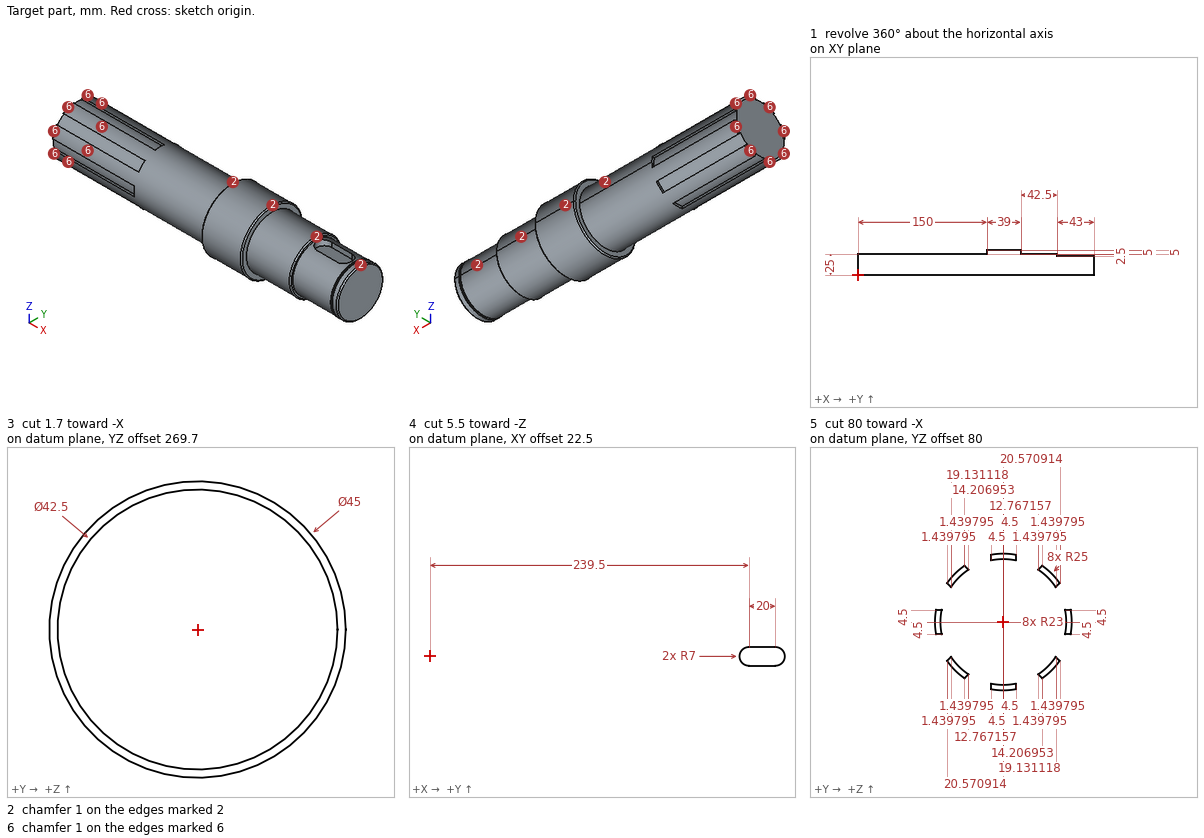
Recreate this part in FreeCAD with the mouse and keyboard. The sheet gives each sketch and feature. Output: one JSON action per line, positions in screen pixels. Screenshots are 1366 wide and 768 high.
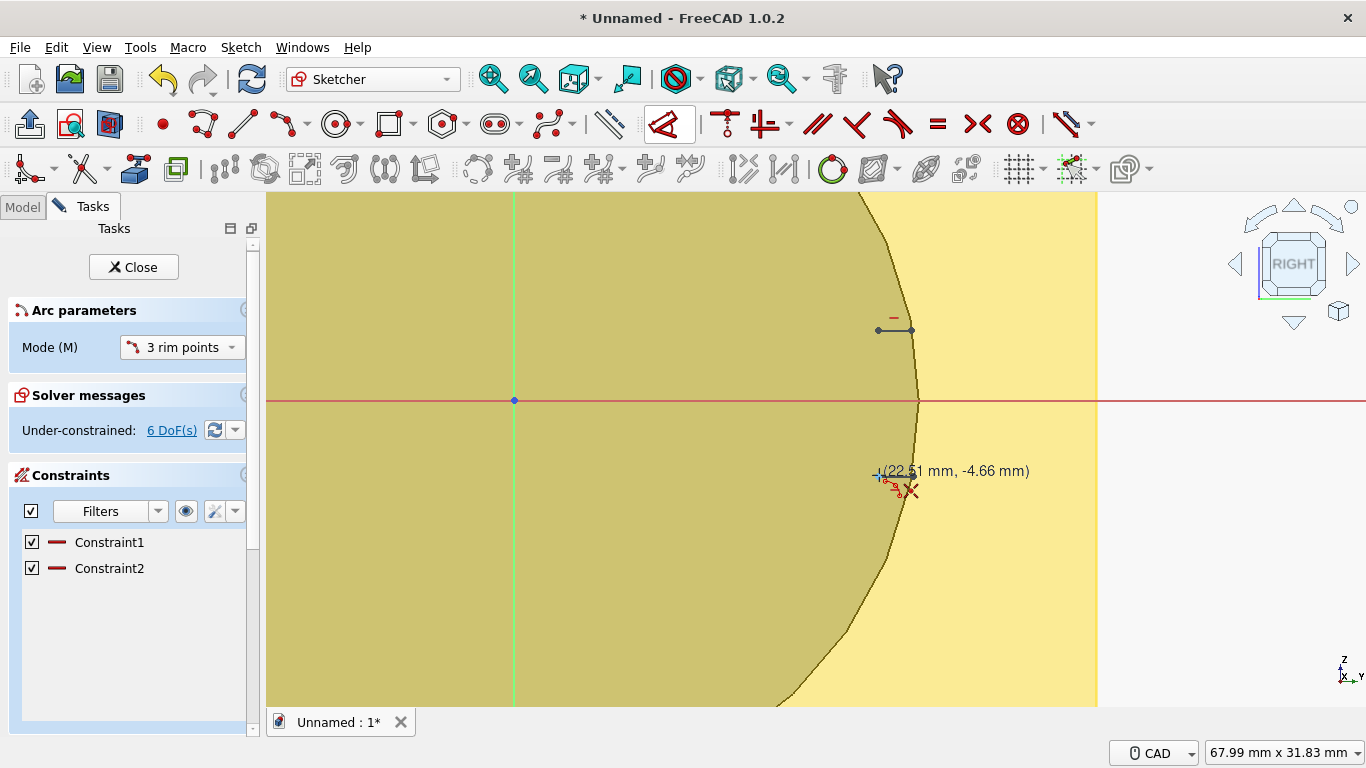
{"action": "left_click", "coordinate": [879, 477]}
{"action": "left_click", "coordinate": [879, 331]}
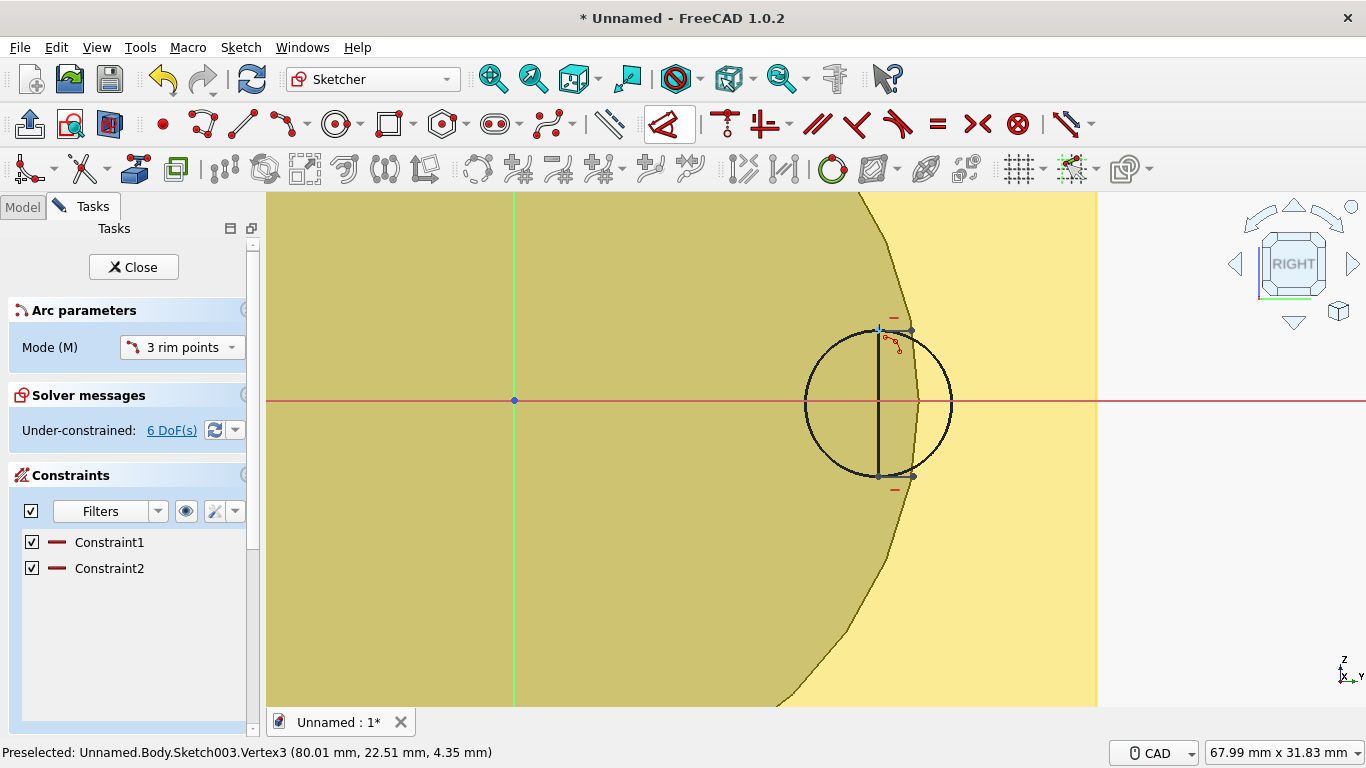
{"action": "scroll", "coordinate": [886, 416], "scroll_direction": "up", "scroll_amount": 5}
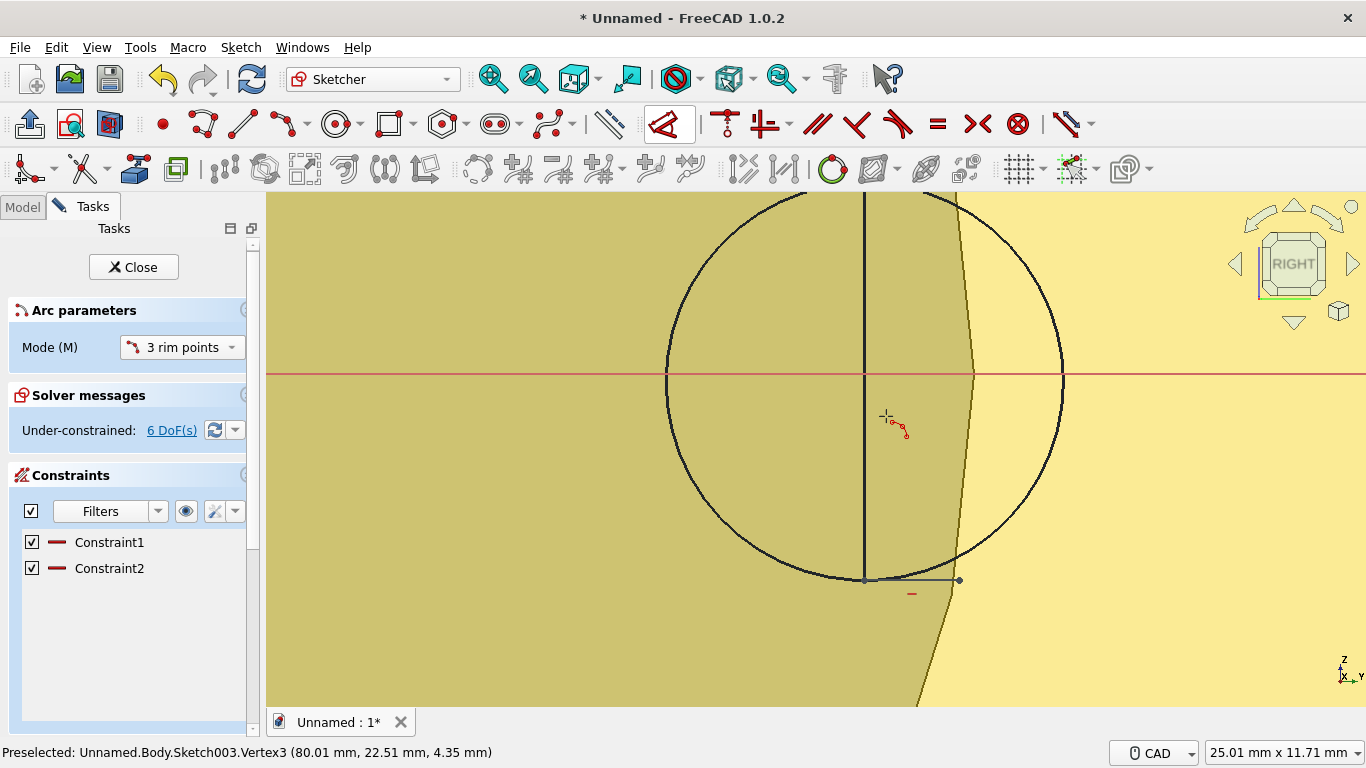
{"action": "left_click", "coordinate": [885, 414]}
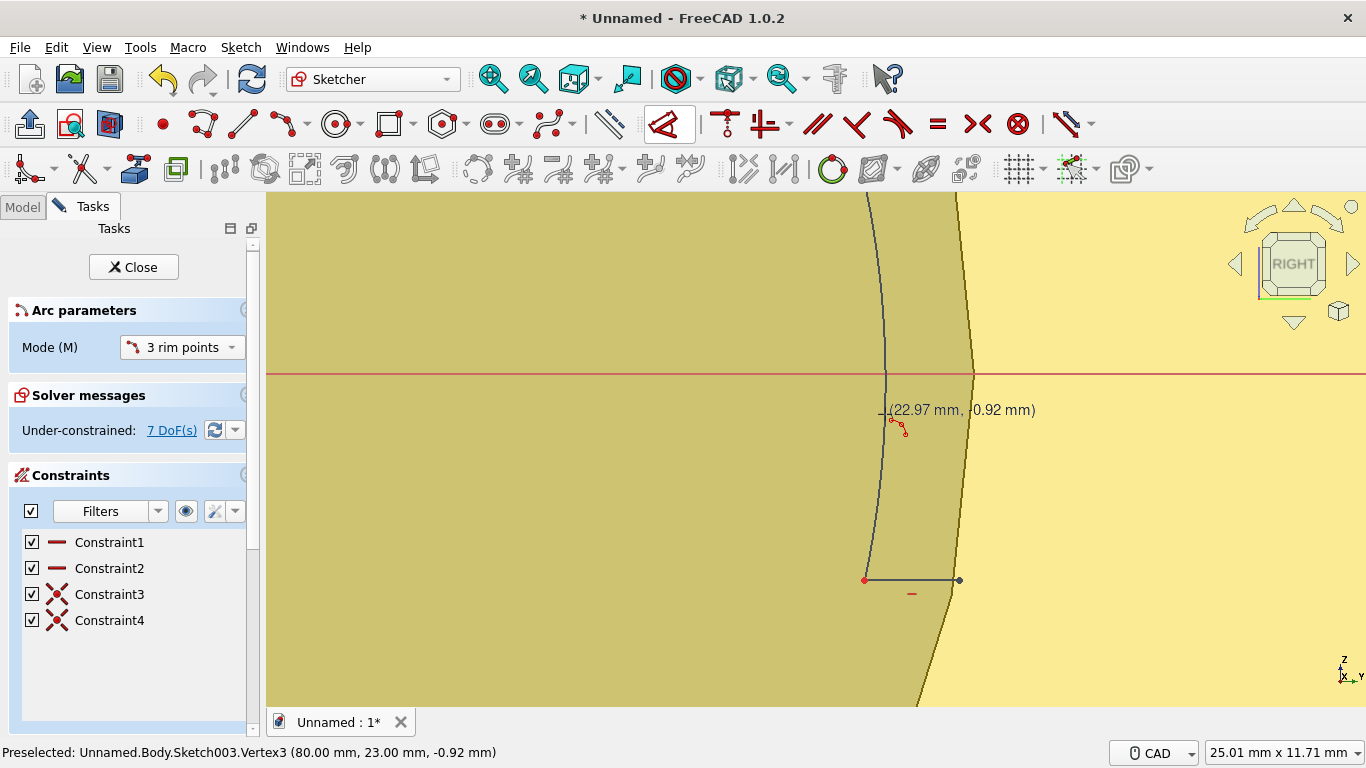
{"action": "scroll", "coordinate": [884, 461], "scroll_direction": "down", "scroll_amount": 10}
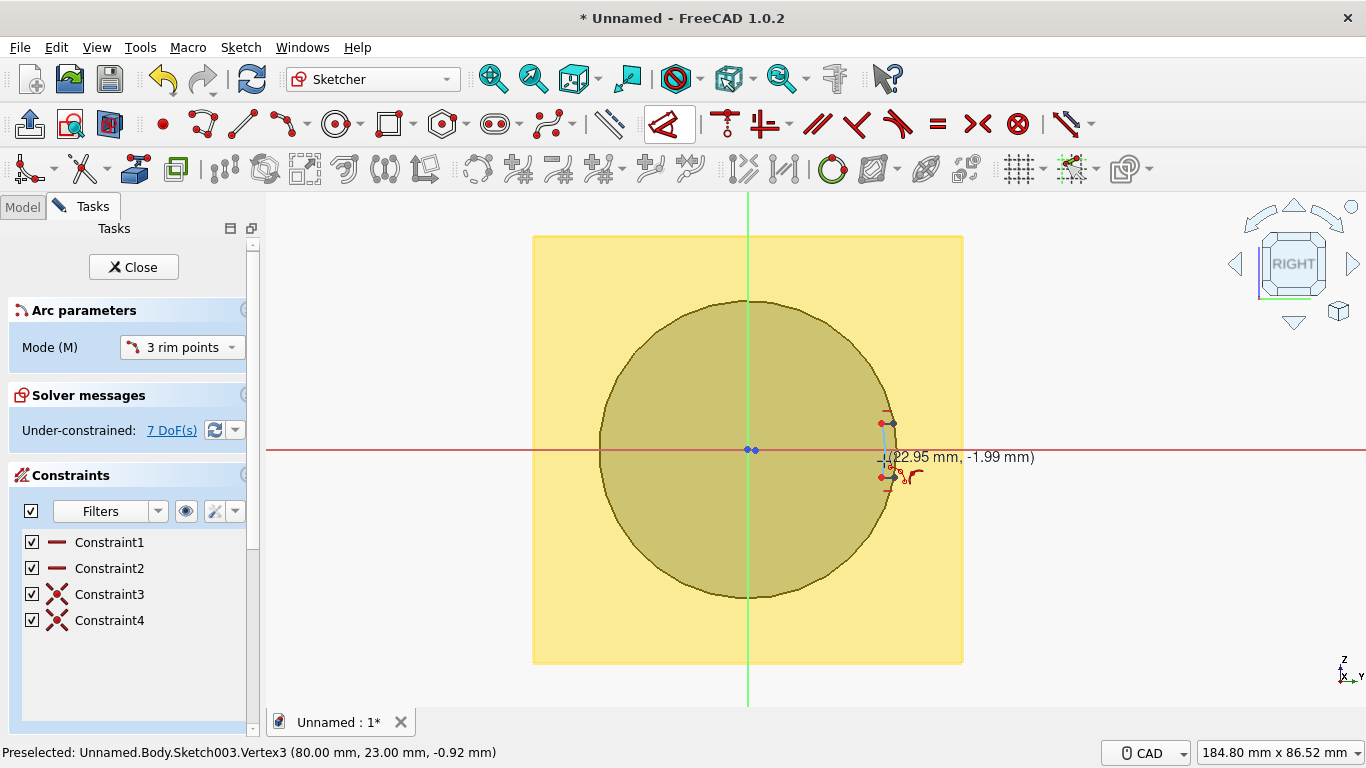
{"action": "scroll", "coordinate": [894, 423], "scroll_direction": "up", "scroll_amount": 5}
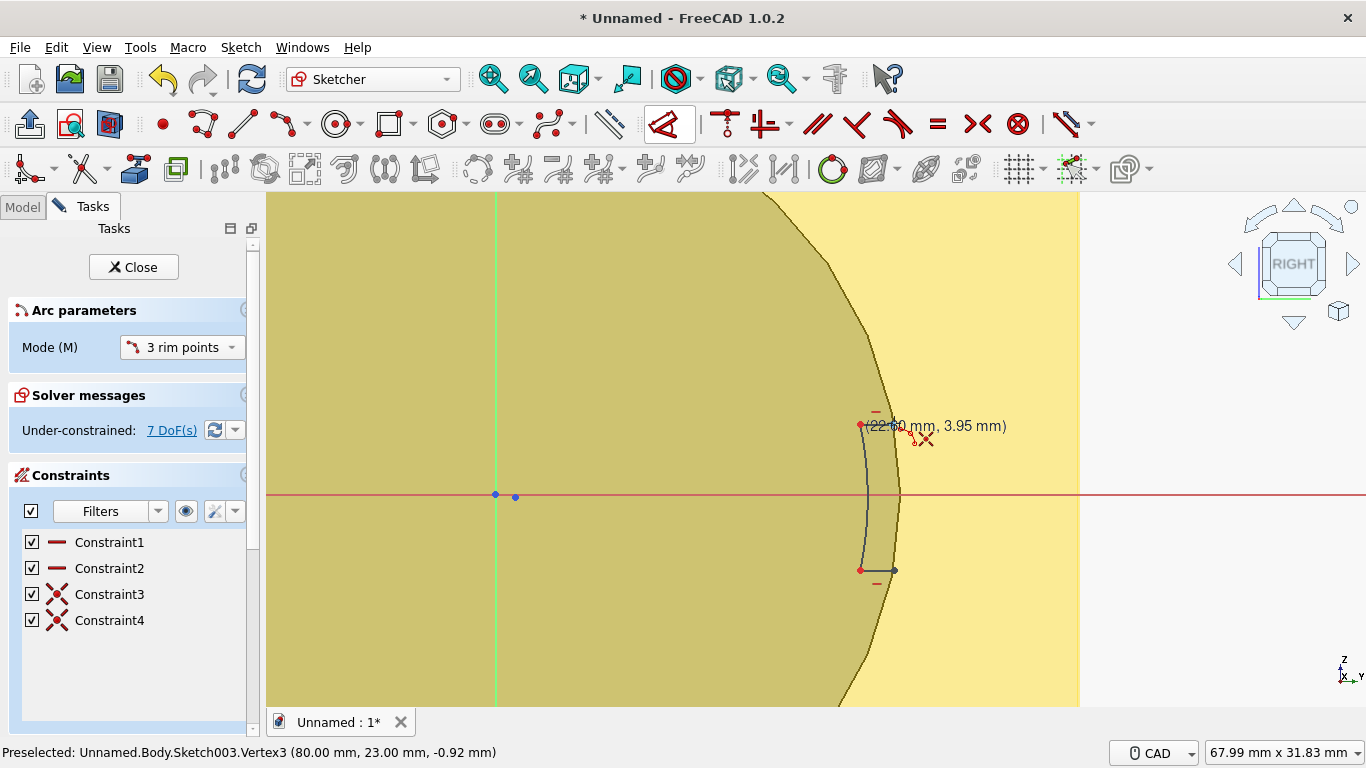
{"action": "left_click", "coordinate": [893, 425]}
{"action": "left_click", "coordinate": [895, 571]}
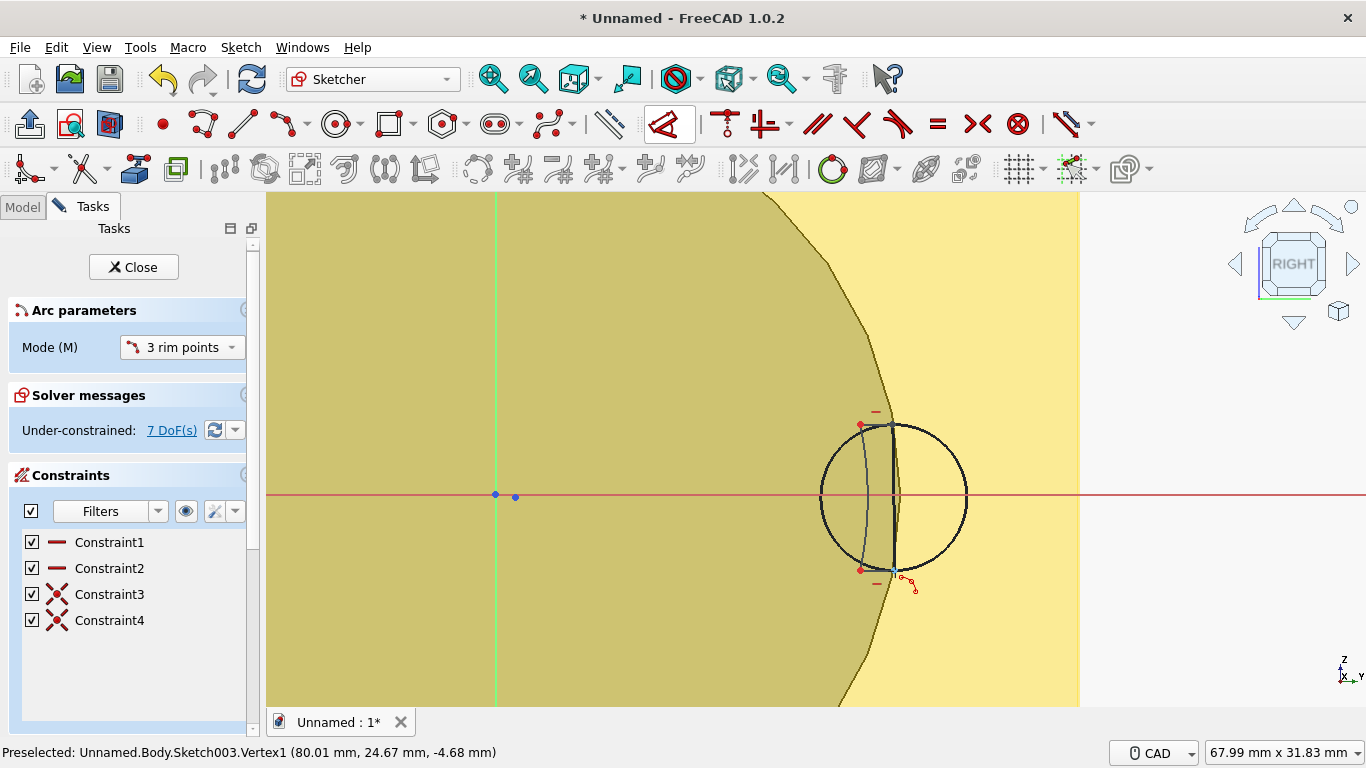
{"action": "scroll", "coordinate": [900, 510], "scroll_direction": "up", "scroll_amount": 5}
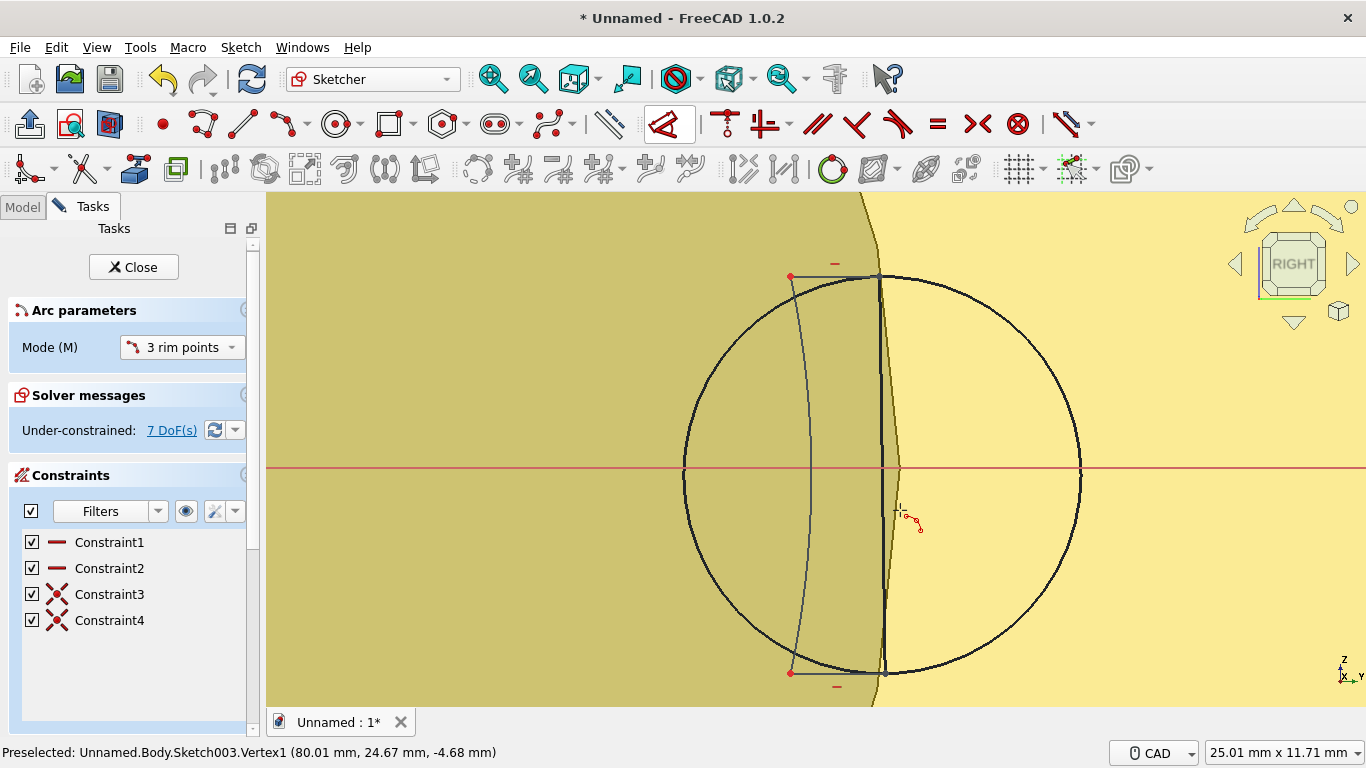
{"action": "left_click", "coordinate": [899, 508]}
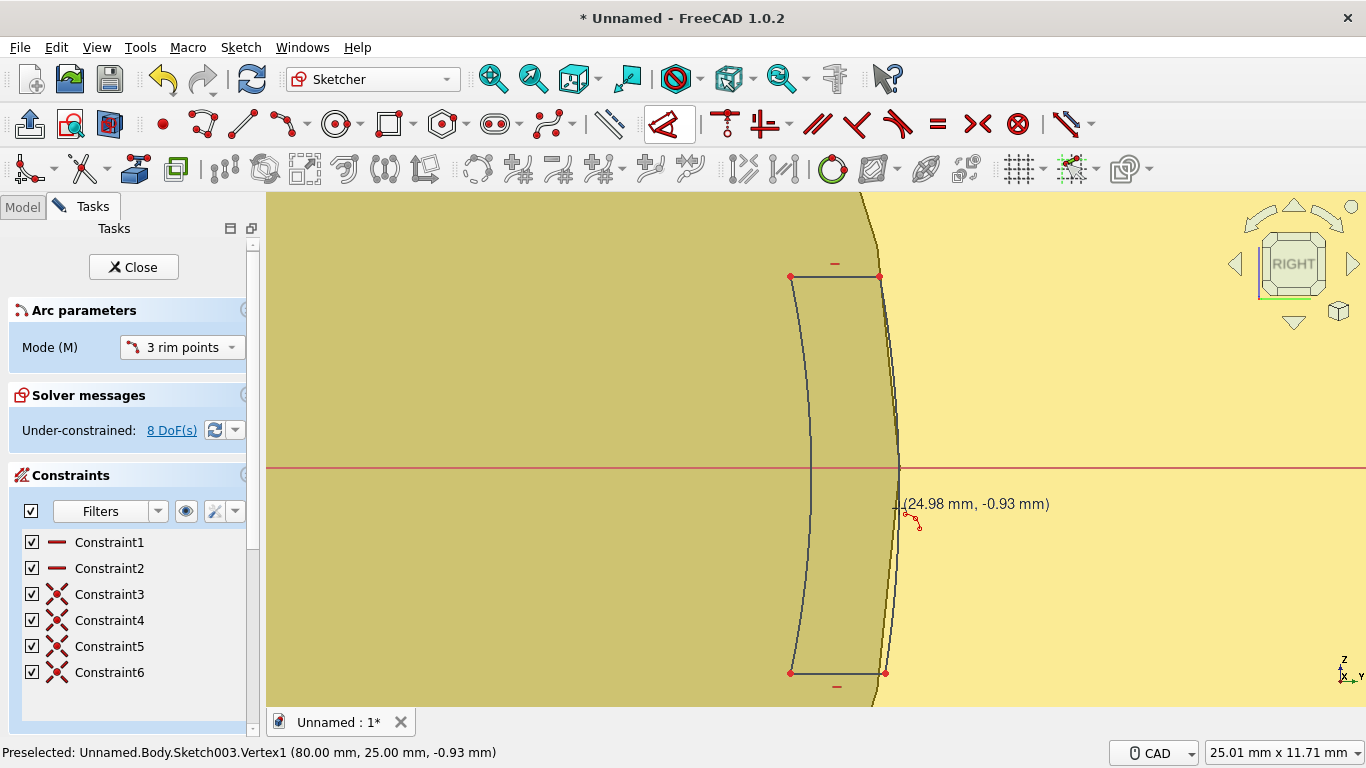
{"action": "left_click", "coordinate": [244, 124]}